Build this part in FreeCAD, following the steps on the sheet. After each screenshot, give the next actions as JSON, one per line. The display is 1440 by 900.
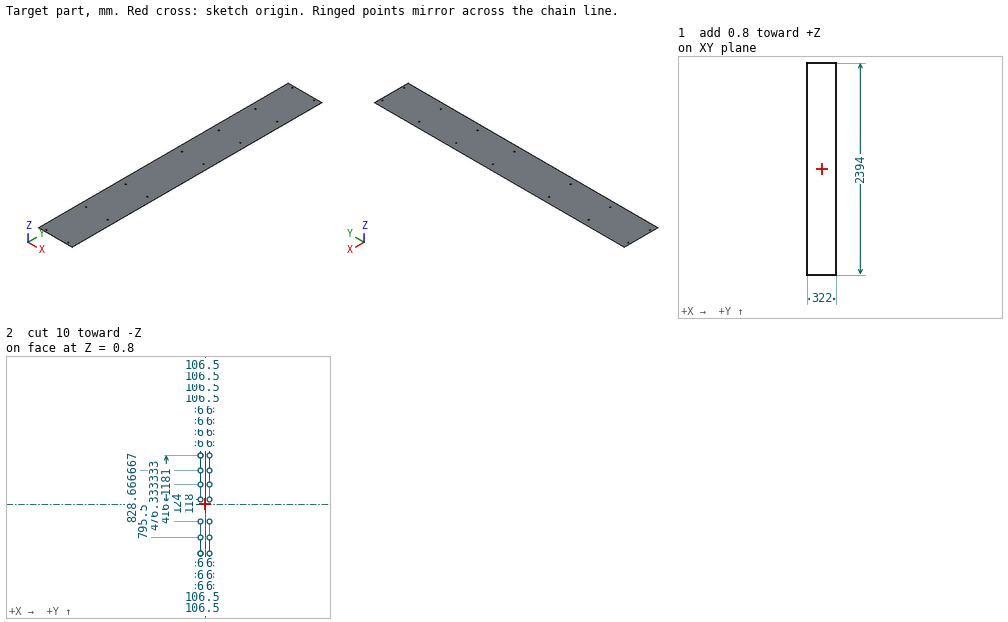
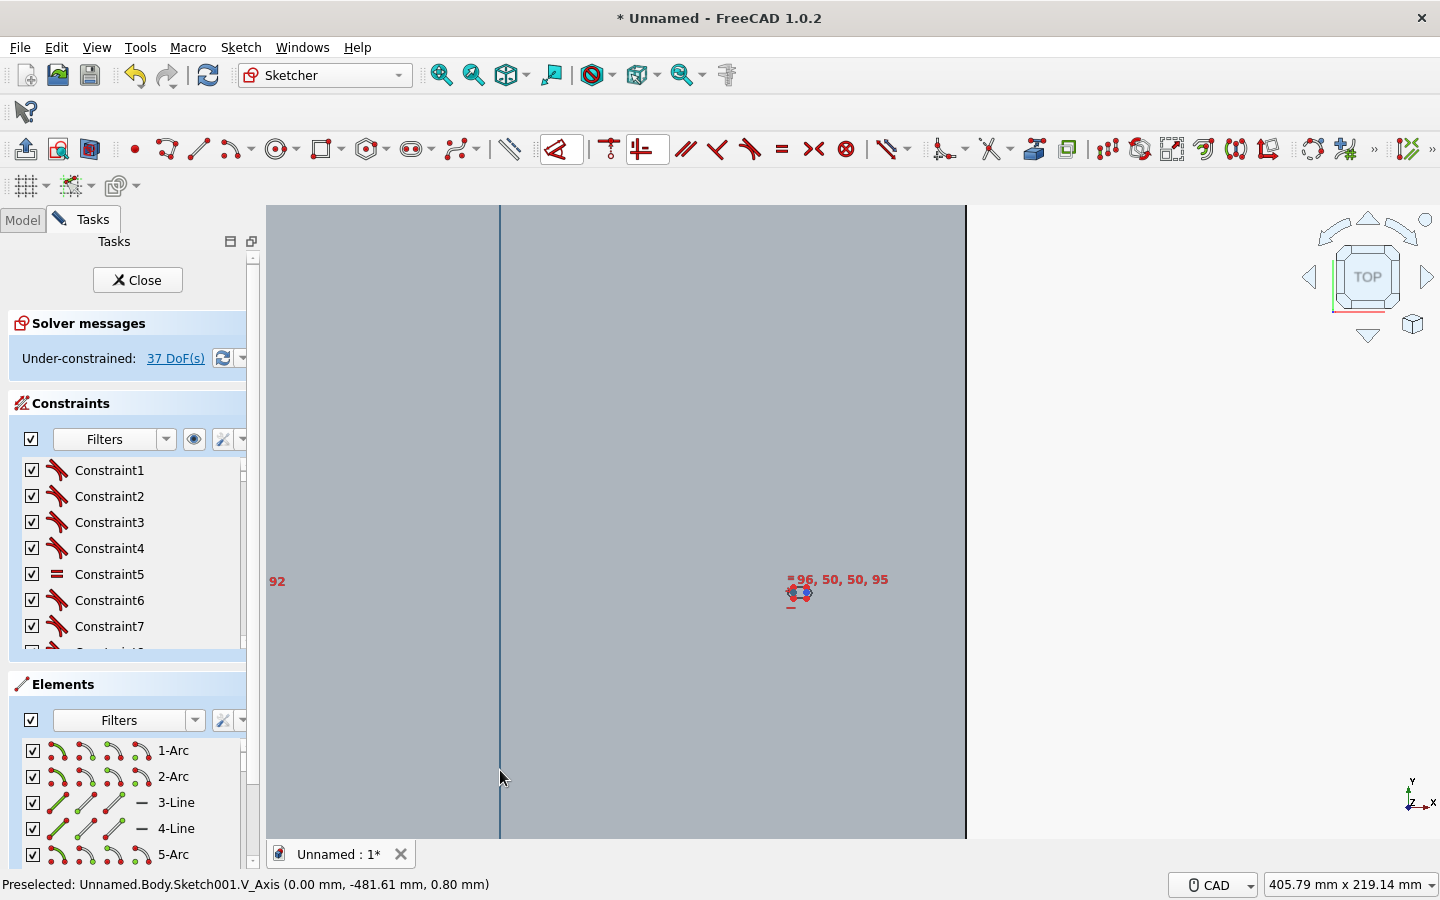
{"action": "left_click", "coordinate": [814, 150]}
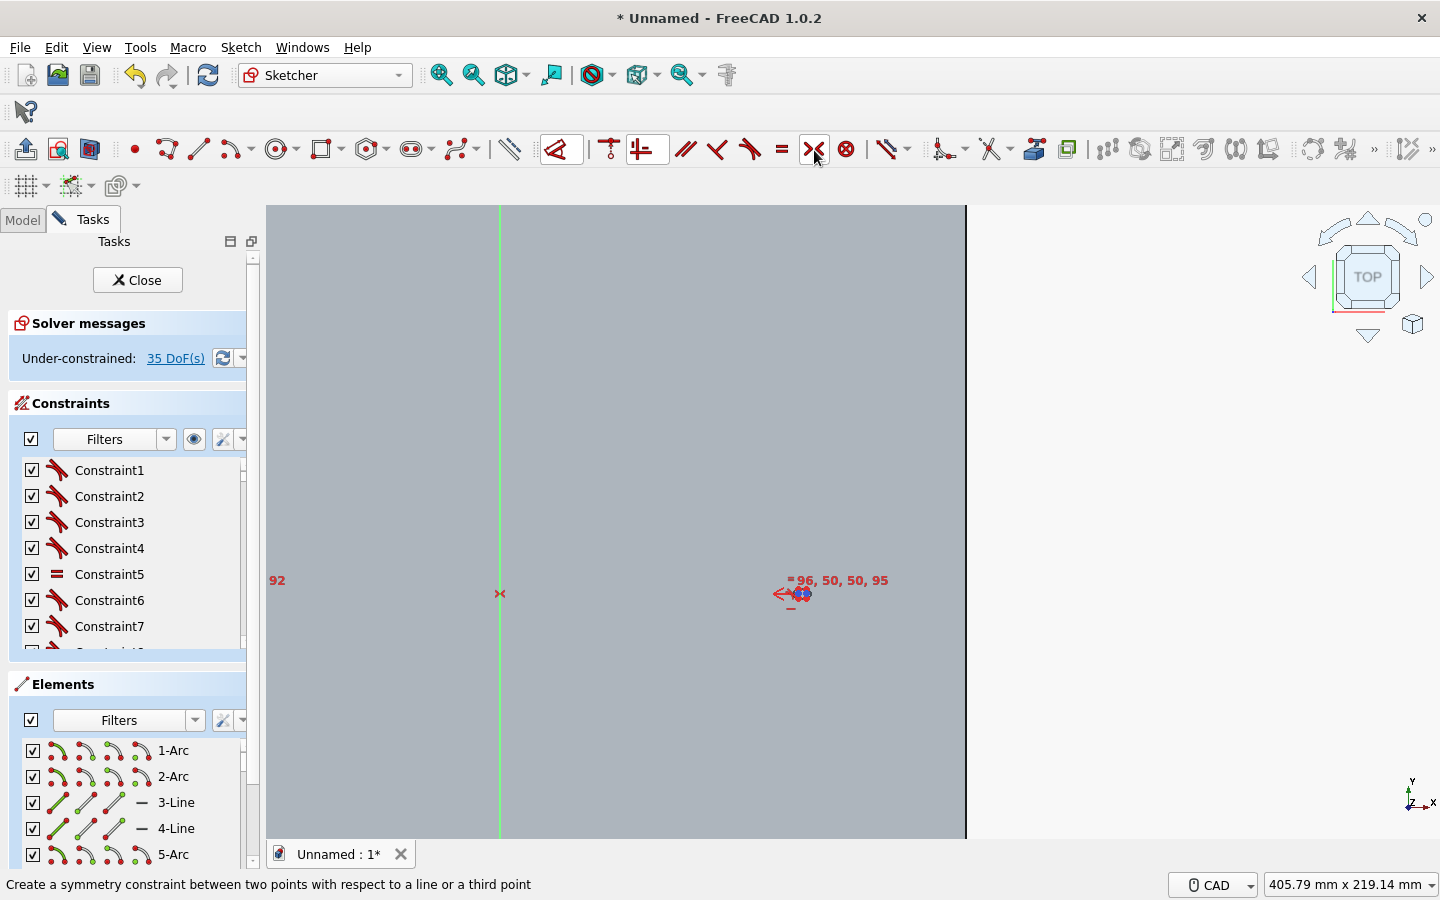
{"action": "scroll", "coordinate": [803, 596], "scroll_direction": "down", "scroll_amount": 14}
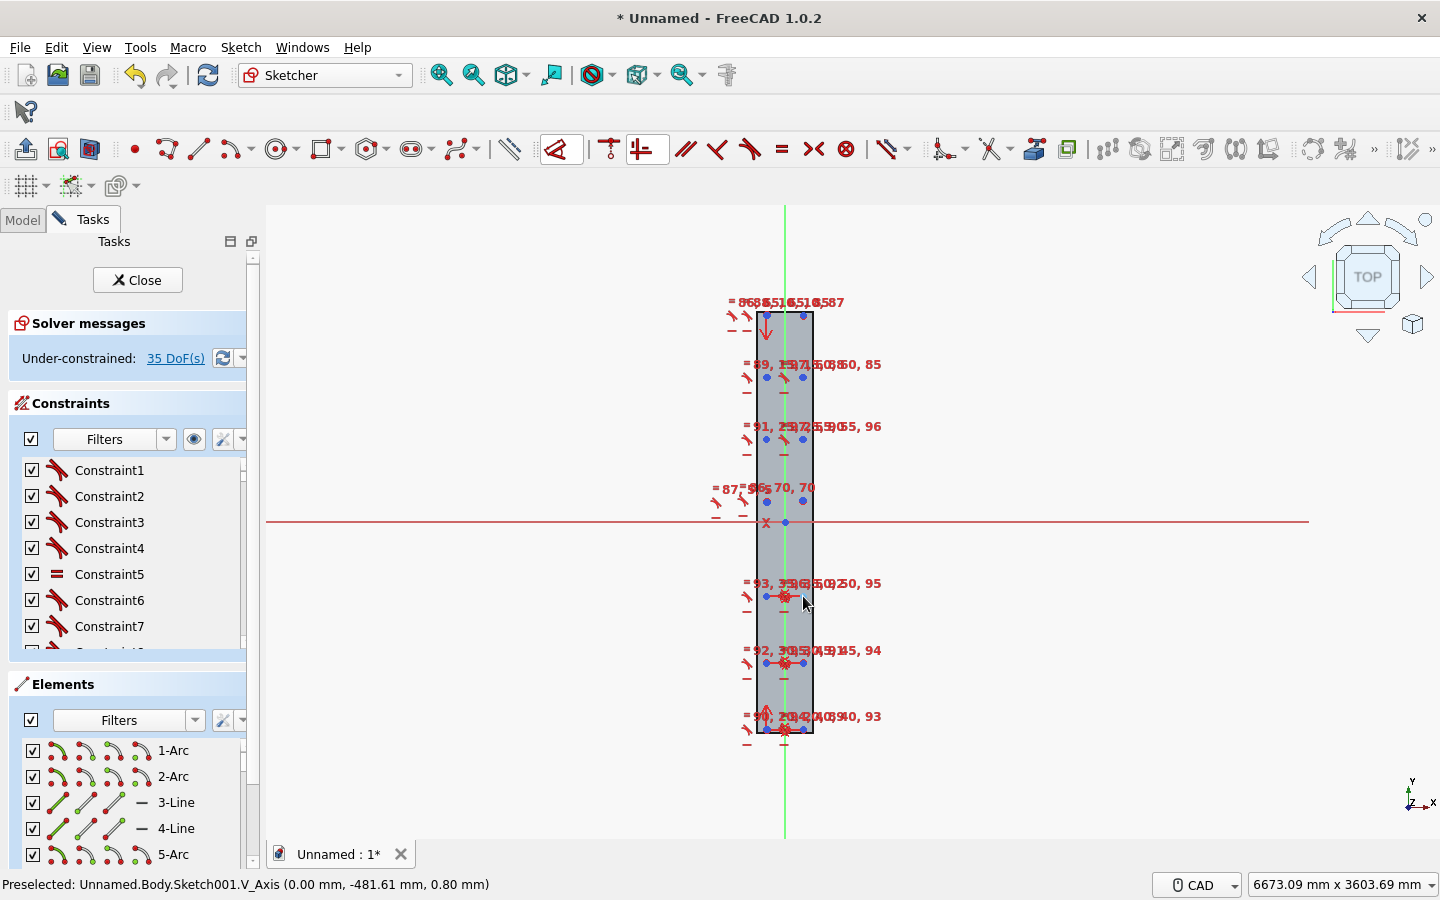
{"action": "scroll", "coordinate": [767, 439], "scroll_direction": "up", "scroll_amount": 14}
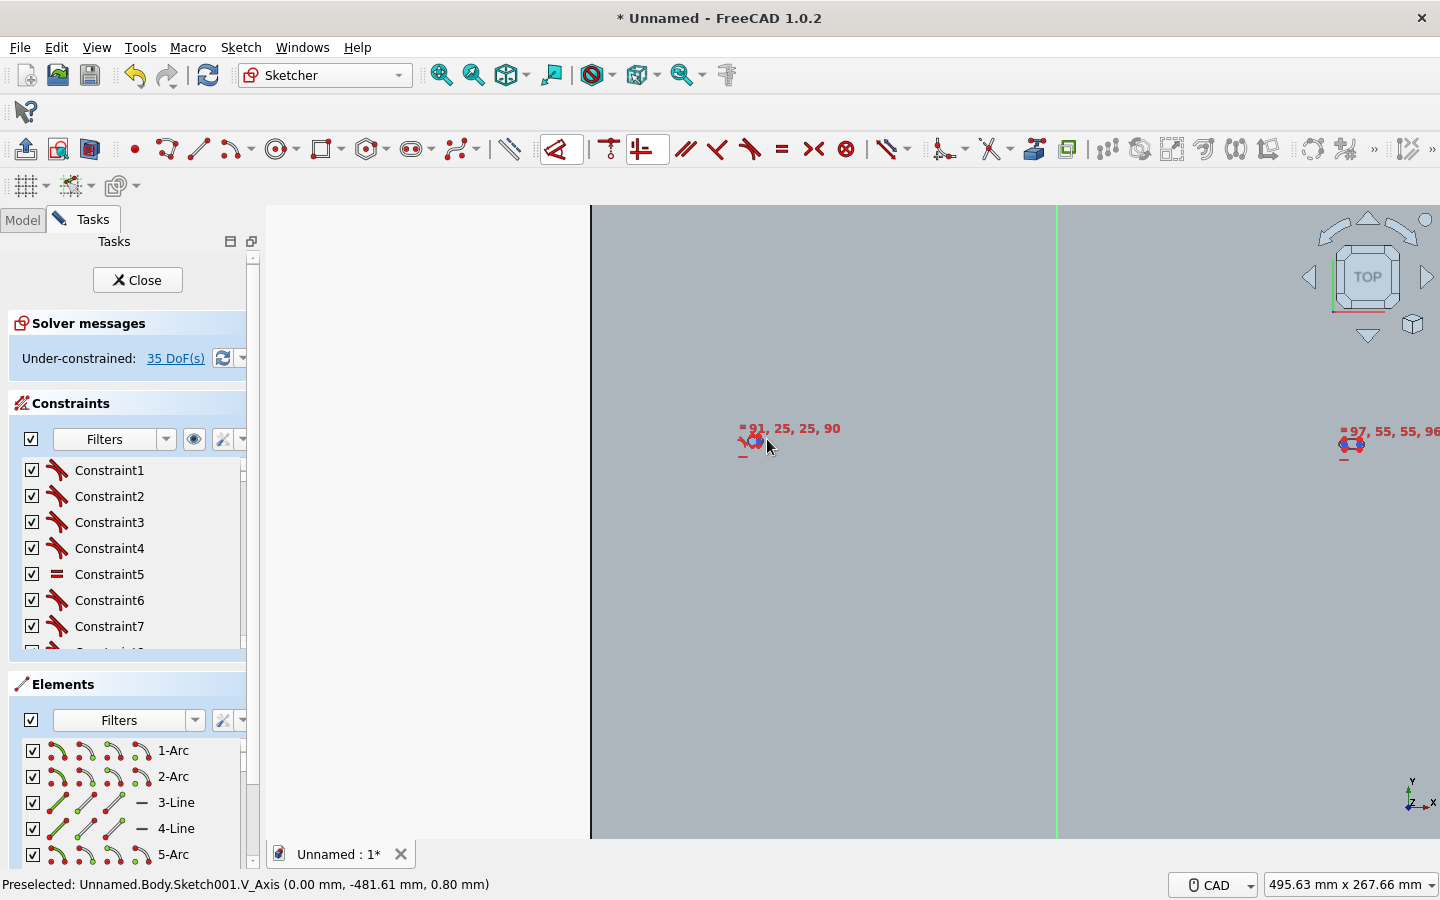
{"action": "left_click", "coordinate": [758, 441]}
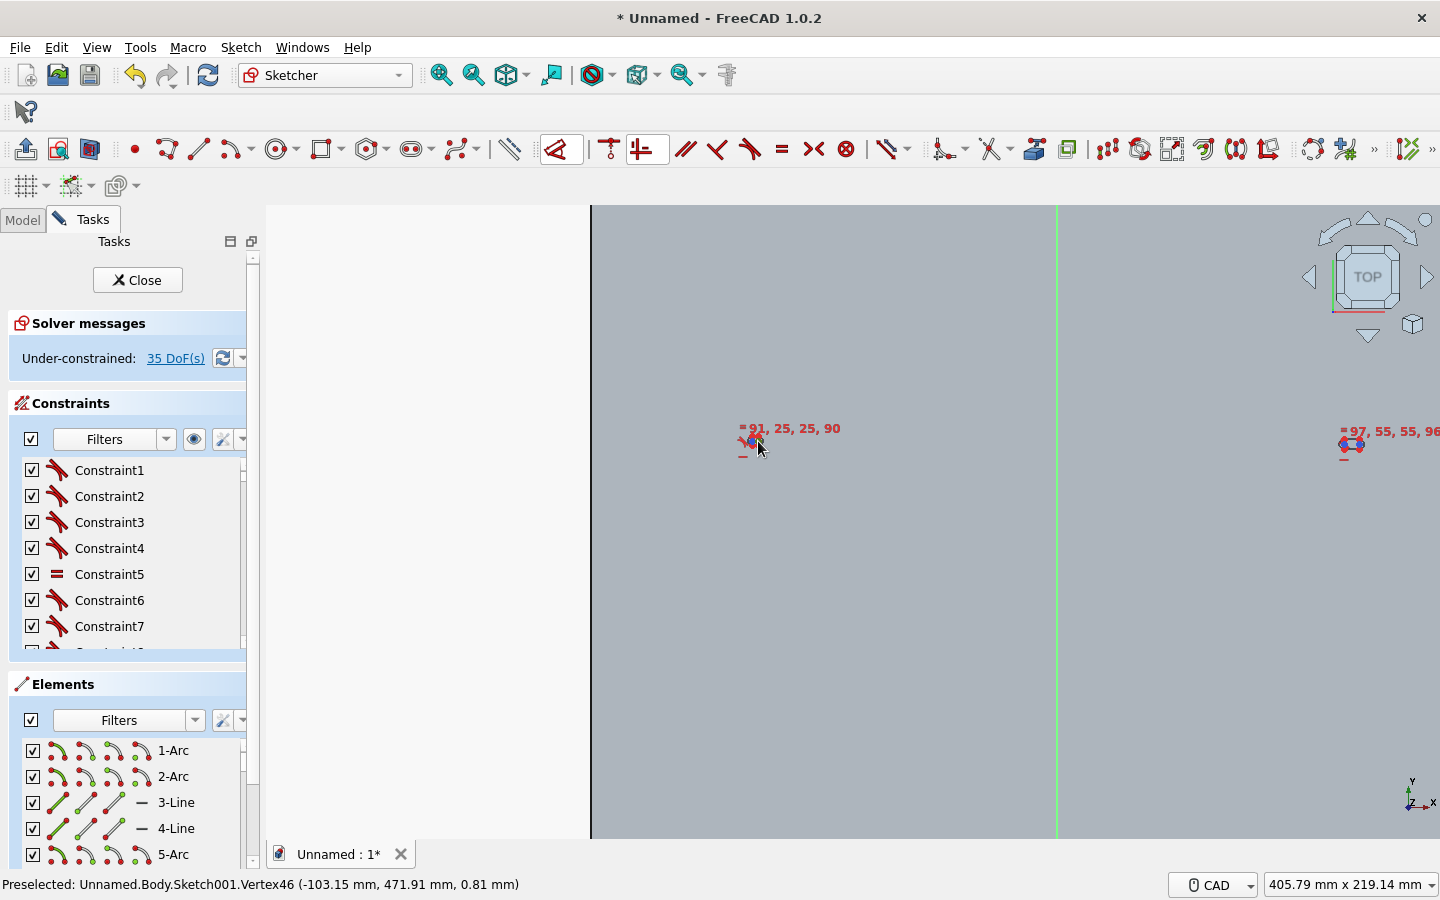
{"action": "scroll", "coordinate": [767, 439], "scroll_direction": "down", "scroll_amount": 14}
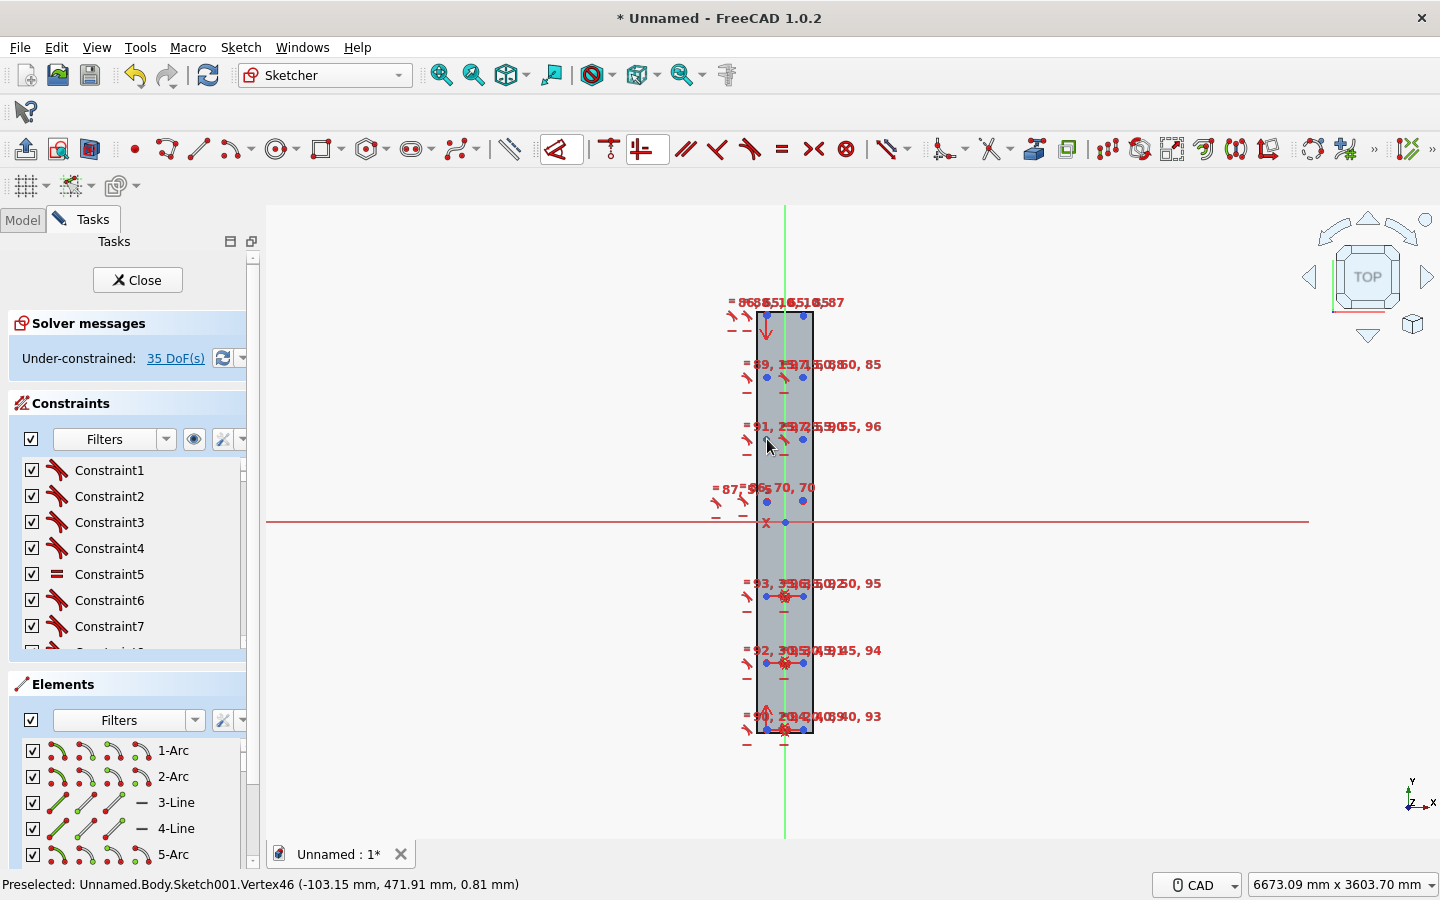
{"action": "scroll", "coordinate": [802, 440], "scroll_direction": "up", "scroll_amount": 14}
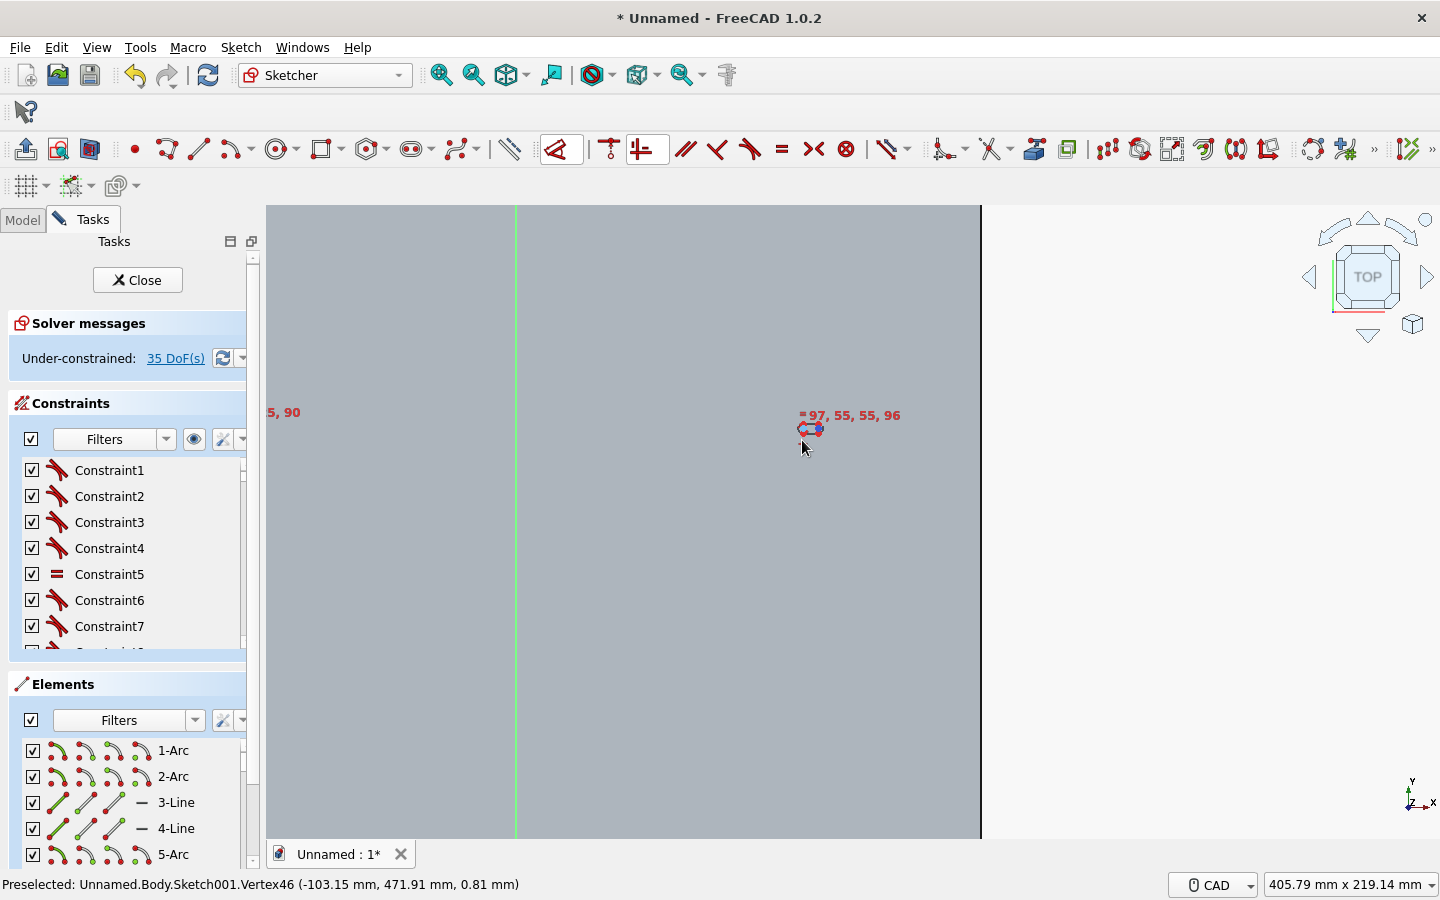
{"action": "left_click", "coordinate": [803, 429]}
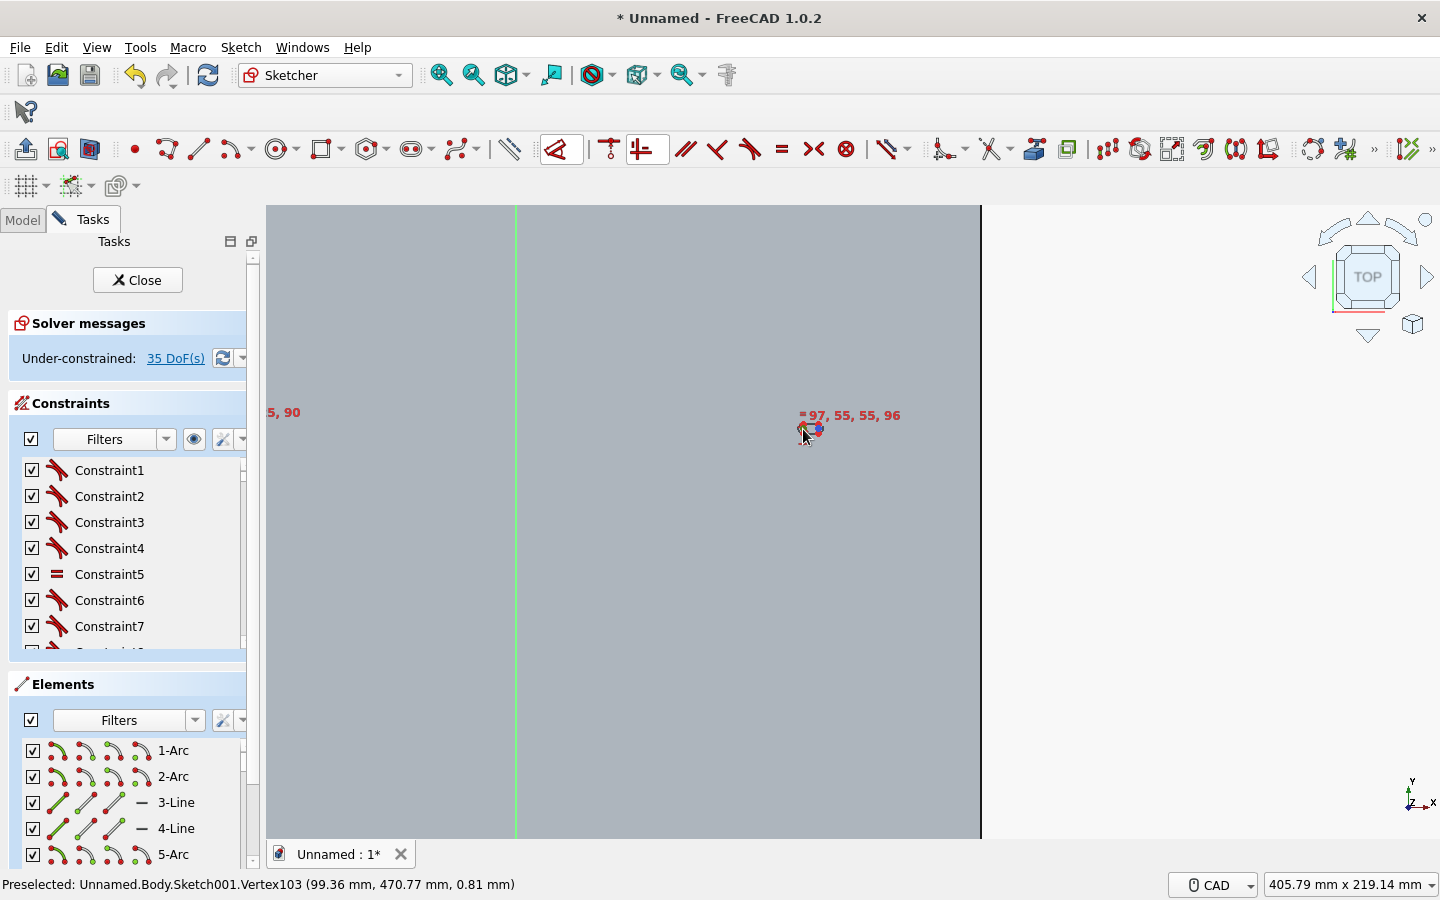
{"action": "left_click", "coordinate": [516, 770]}